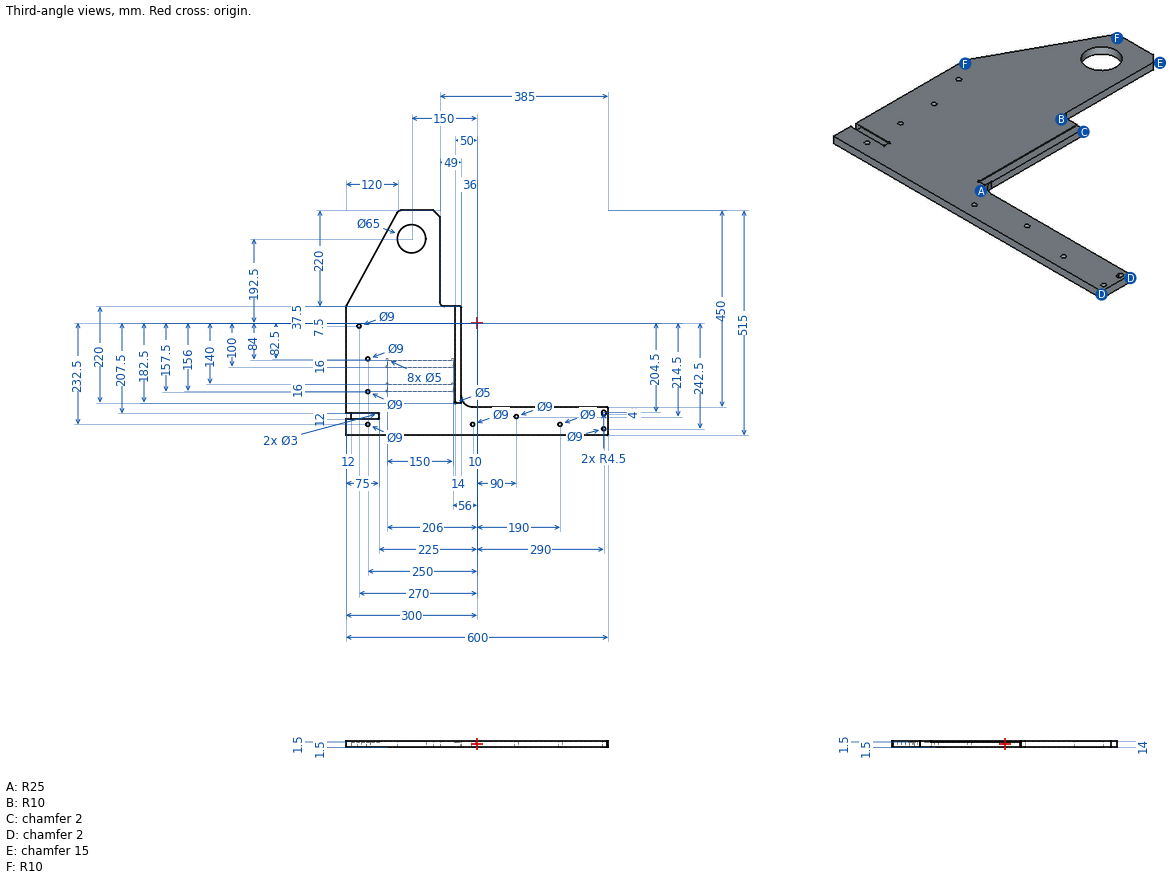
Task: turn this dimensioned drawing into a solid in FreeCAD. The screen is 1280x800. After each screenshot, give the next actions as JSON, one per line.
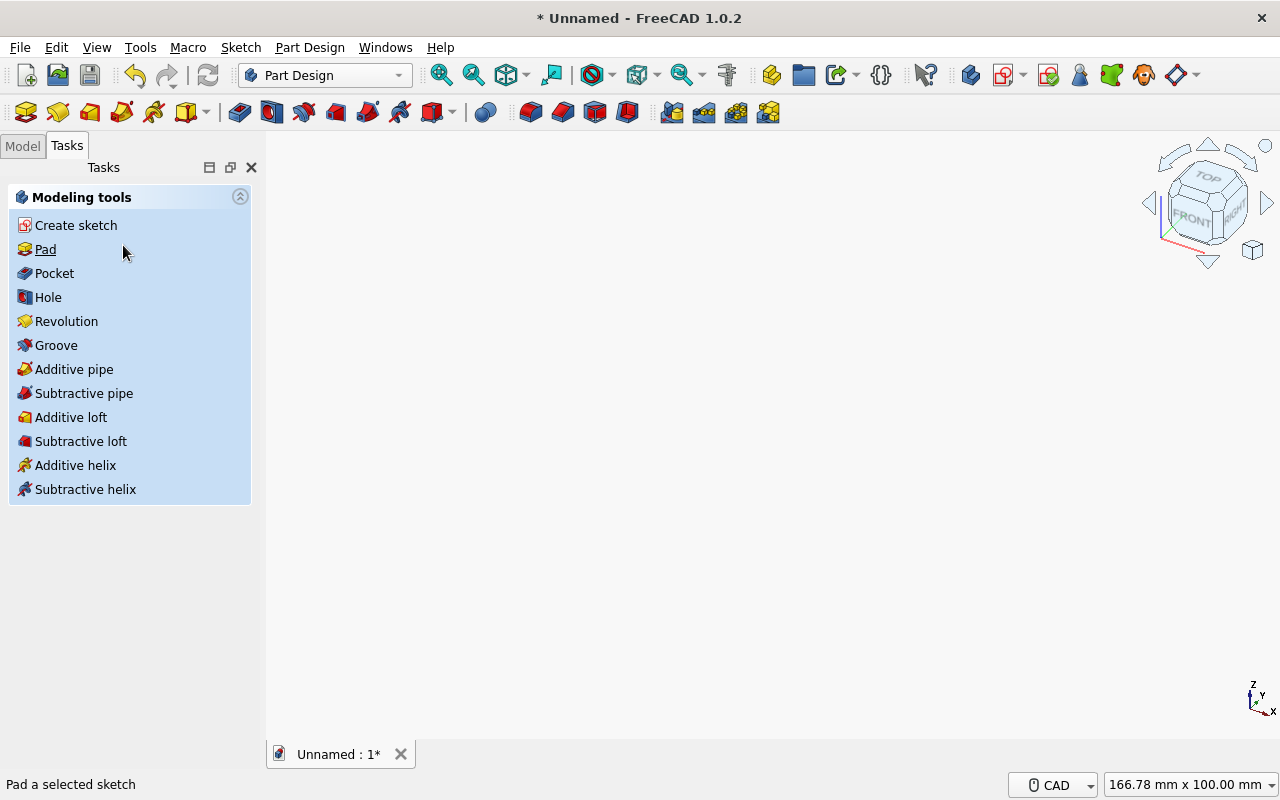
{"action": "left_click", "coordinate": [26, 112]}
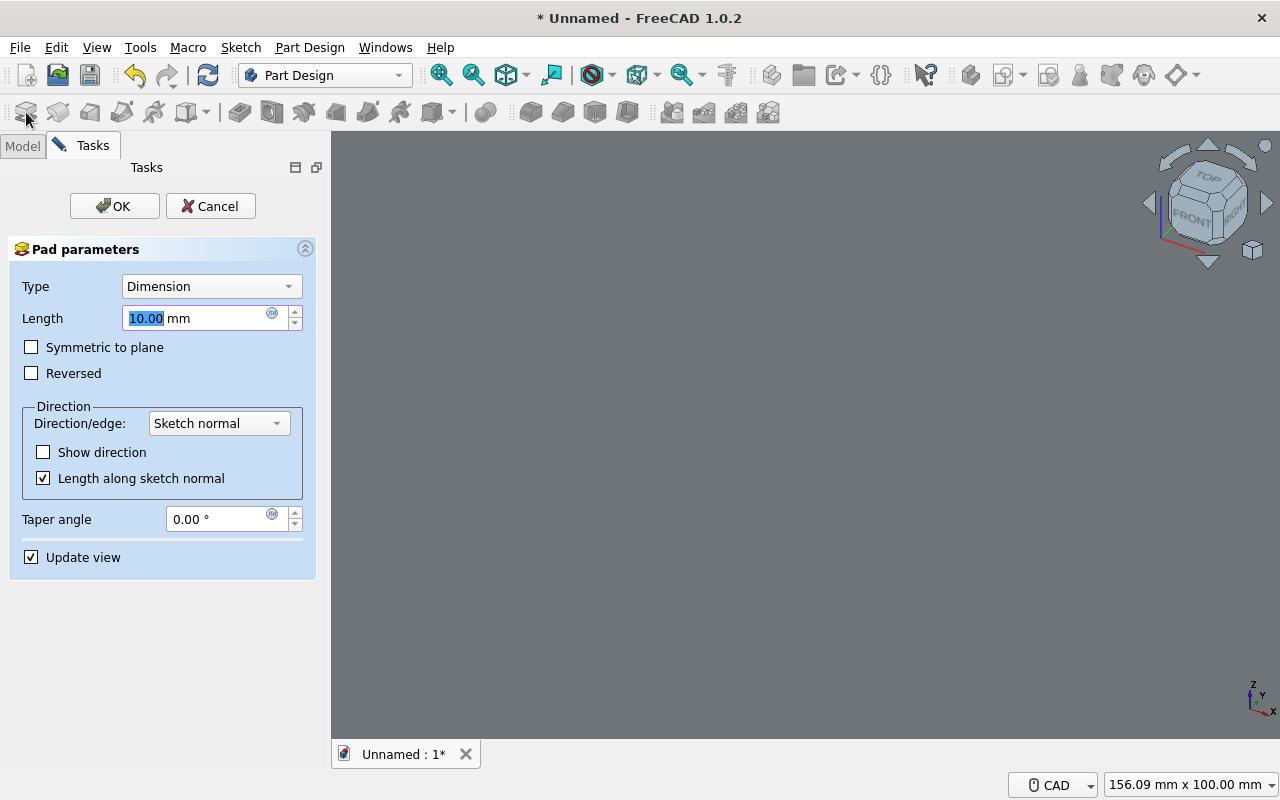
{"action": "type", "text": "14"}
{"action": "key", "text": "Tab"}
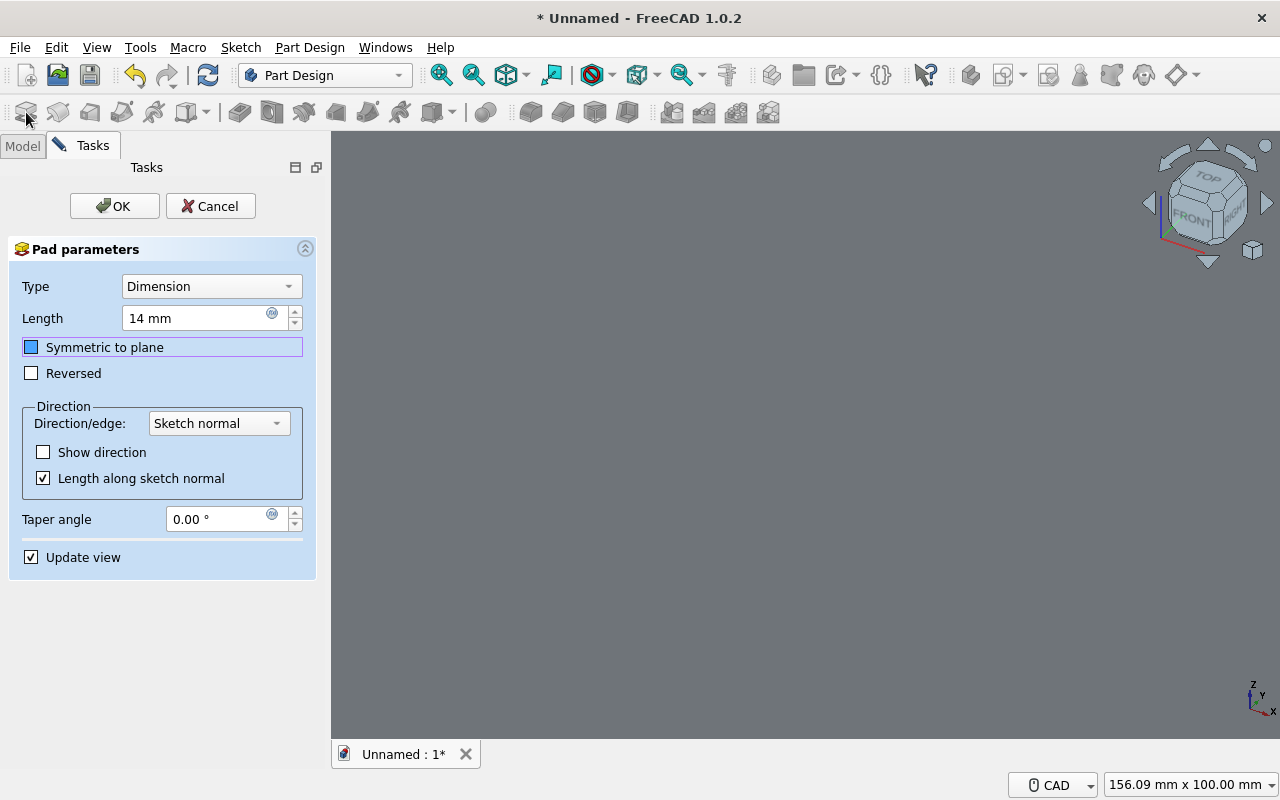
{"action": "left_click", "coordinate": [30, 347]}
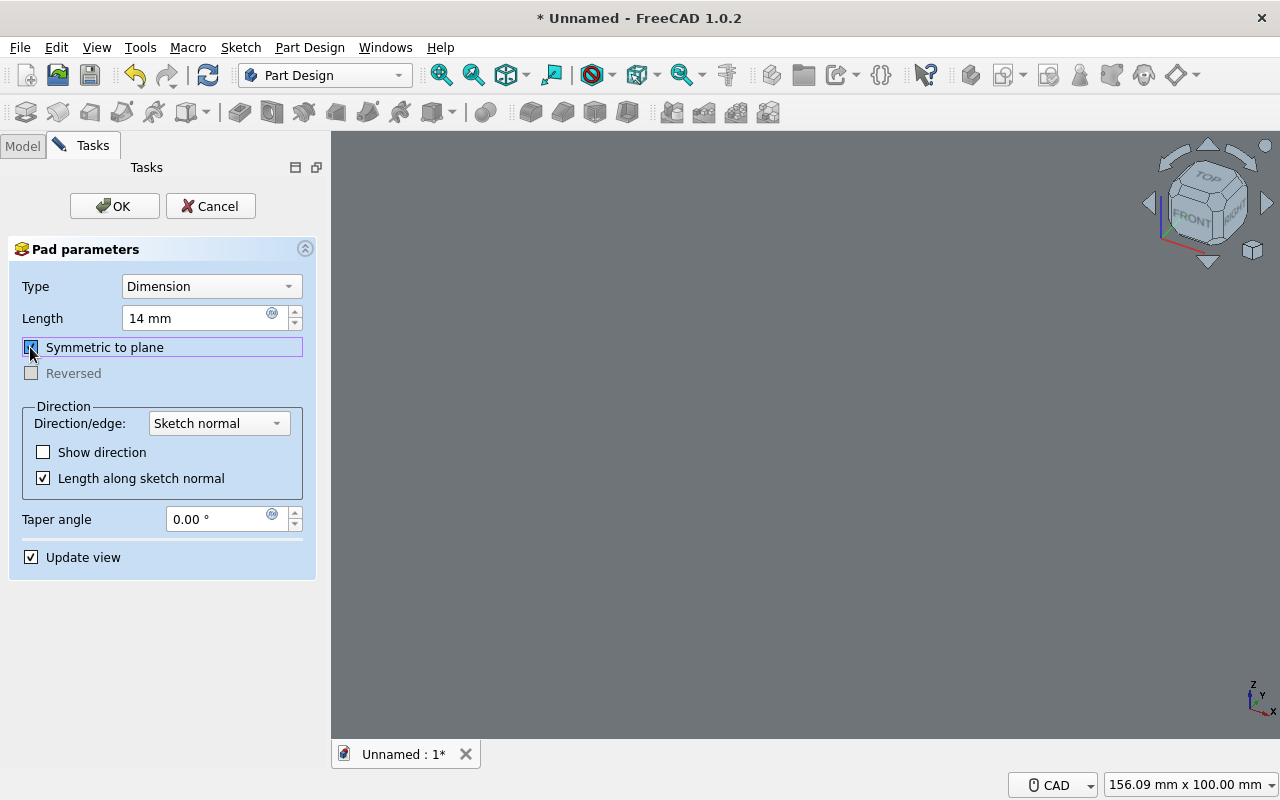
{"action": "left_click", "coordinate": [115, 206]}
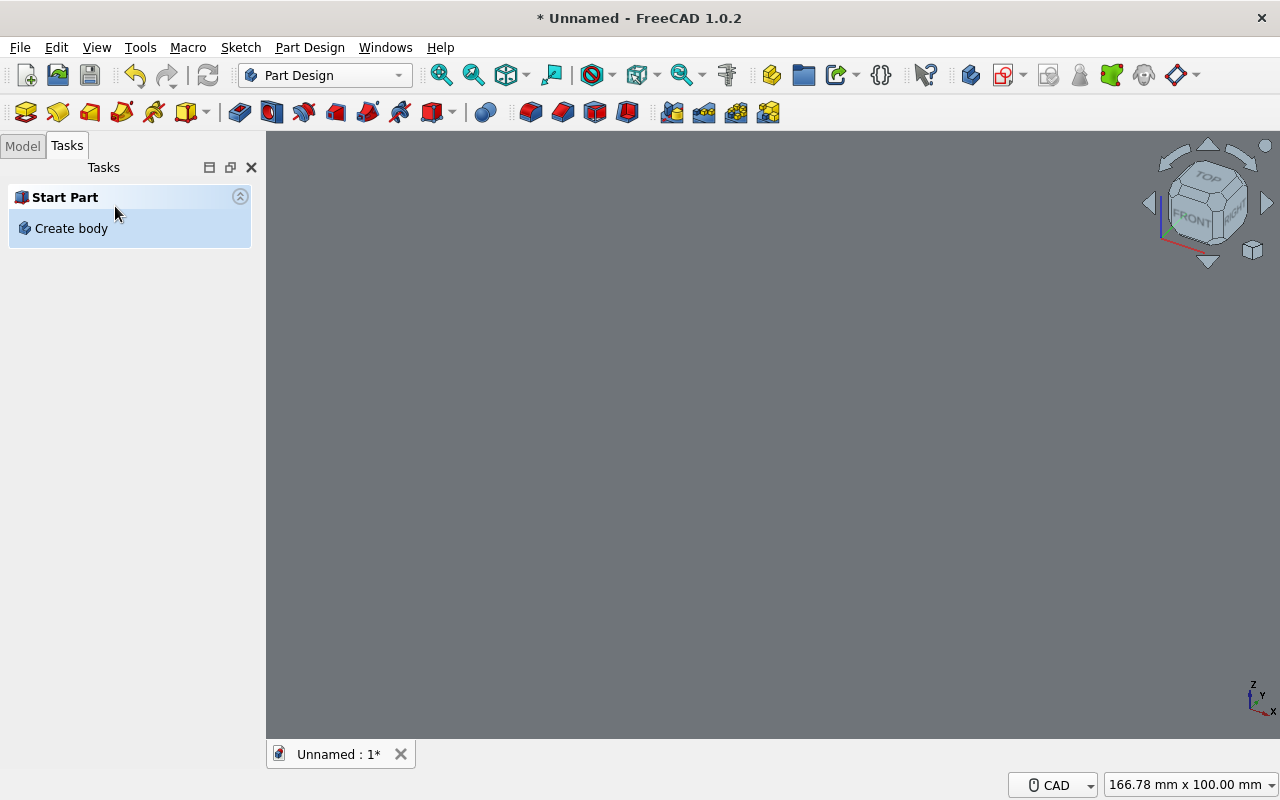
{"action": "left_click", "coordinate": [442, 76]}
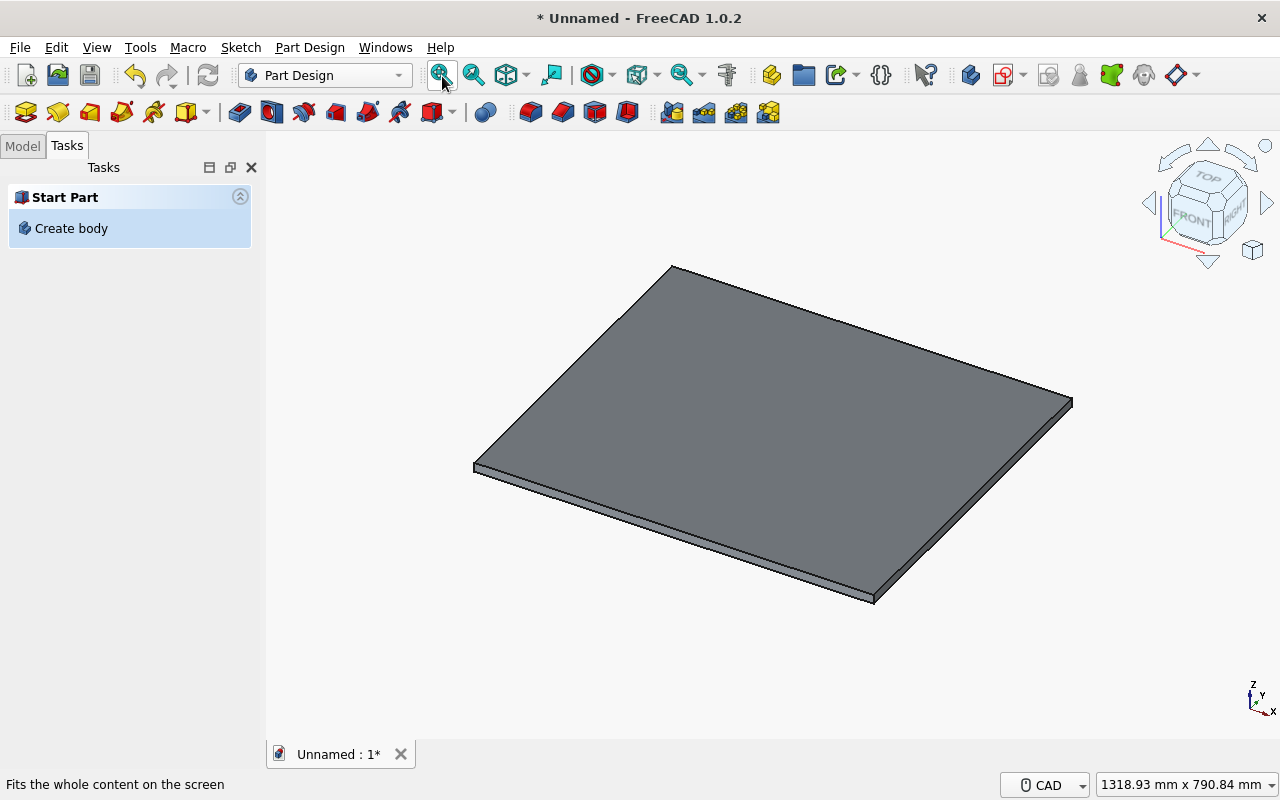
{"action": "left_click", "coordinate": [773, 430]}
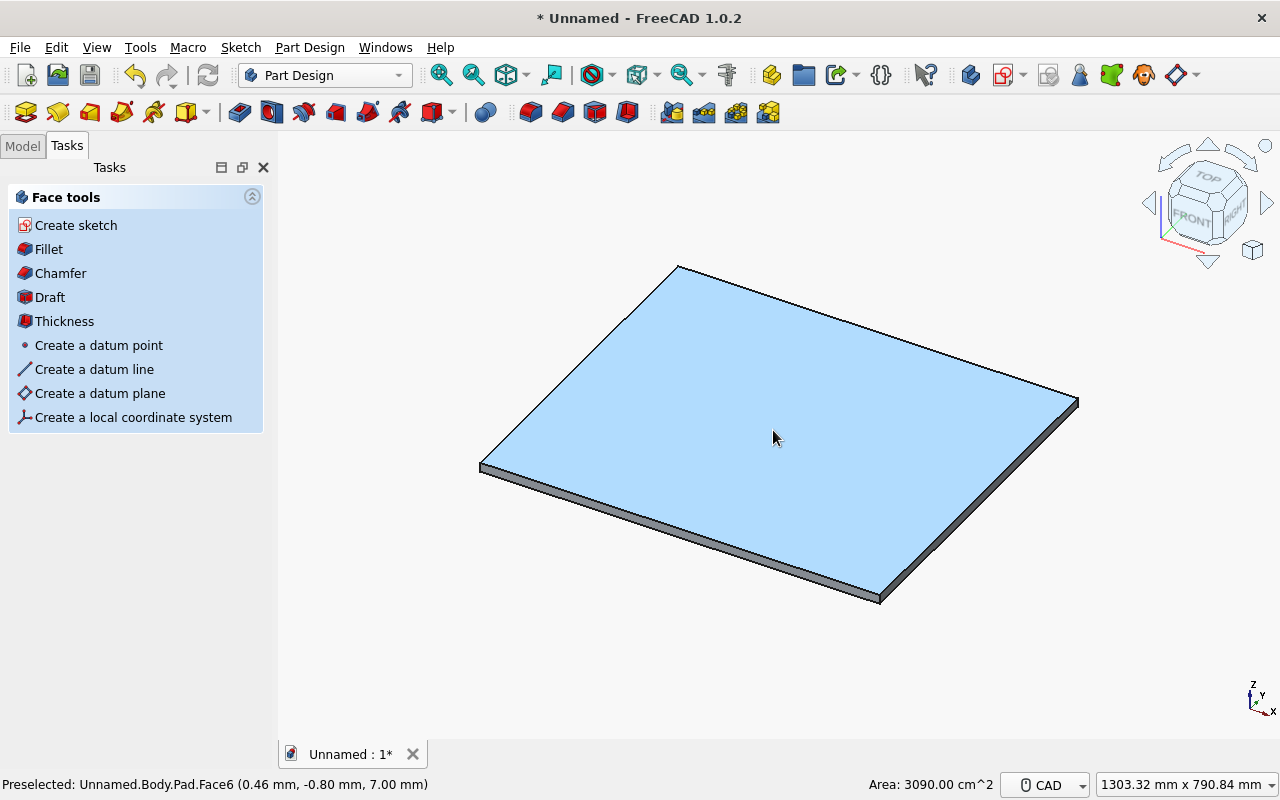
{"action": "left_click", "coordinate": [1004, 76]}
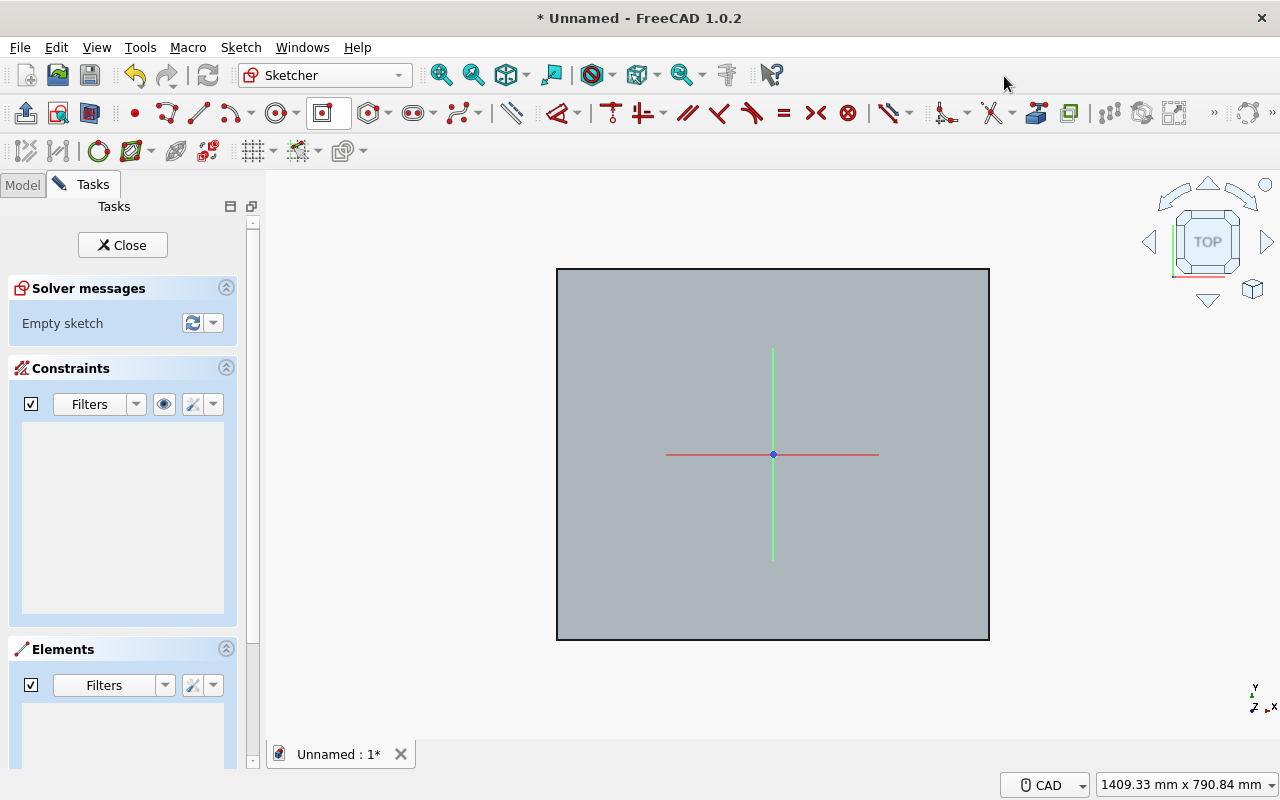
{"action": "scroll", "coordinate": [659, 294], "scroll_direction": "up", "scroll_amount": 10}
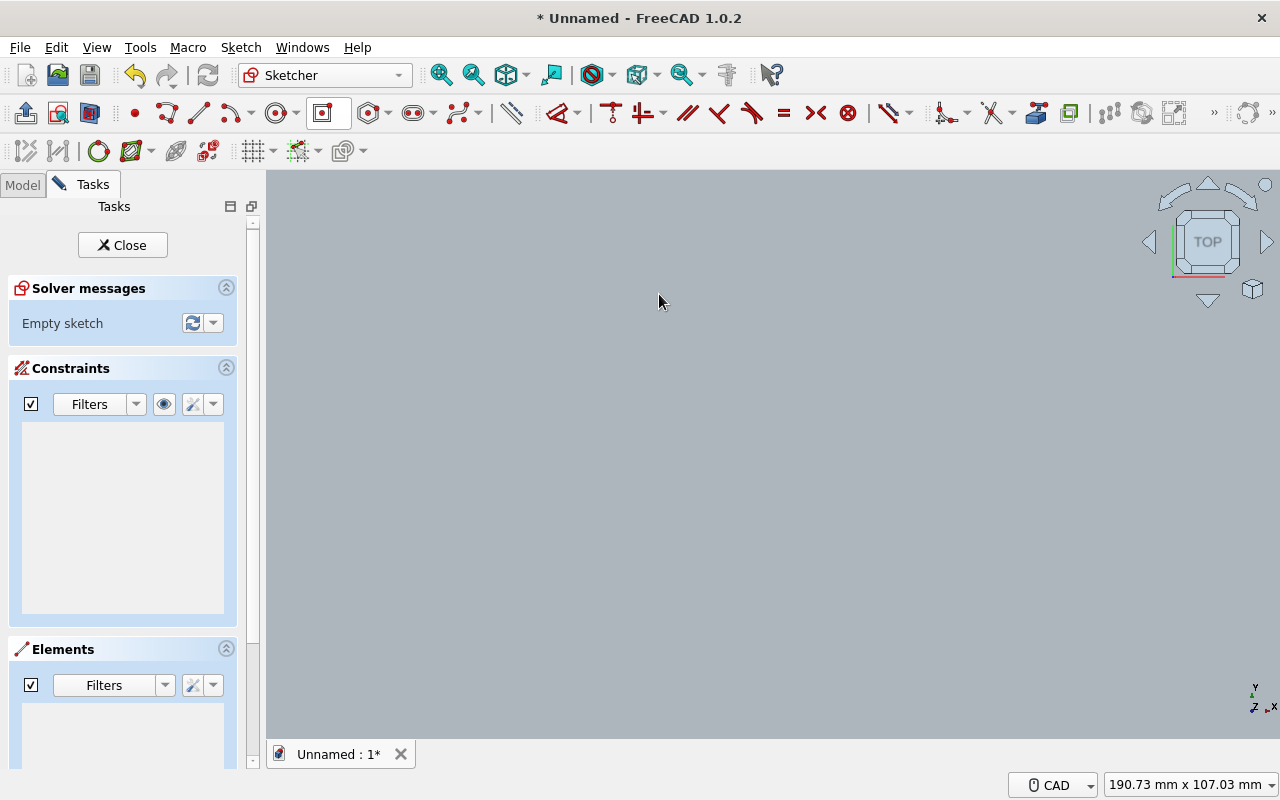
{"action": "left_click", "coordinate": [276, 114]}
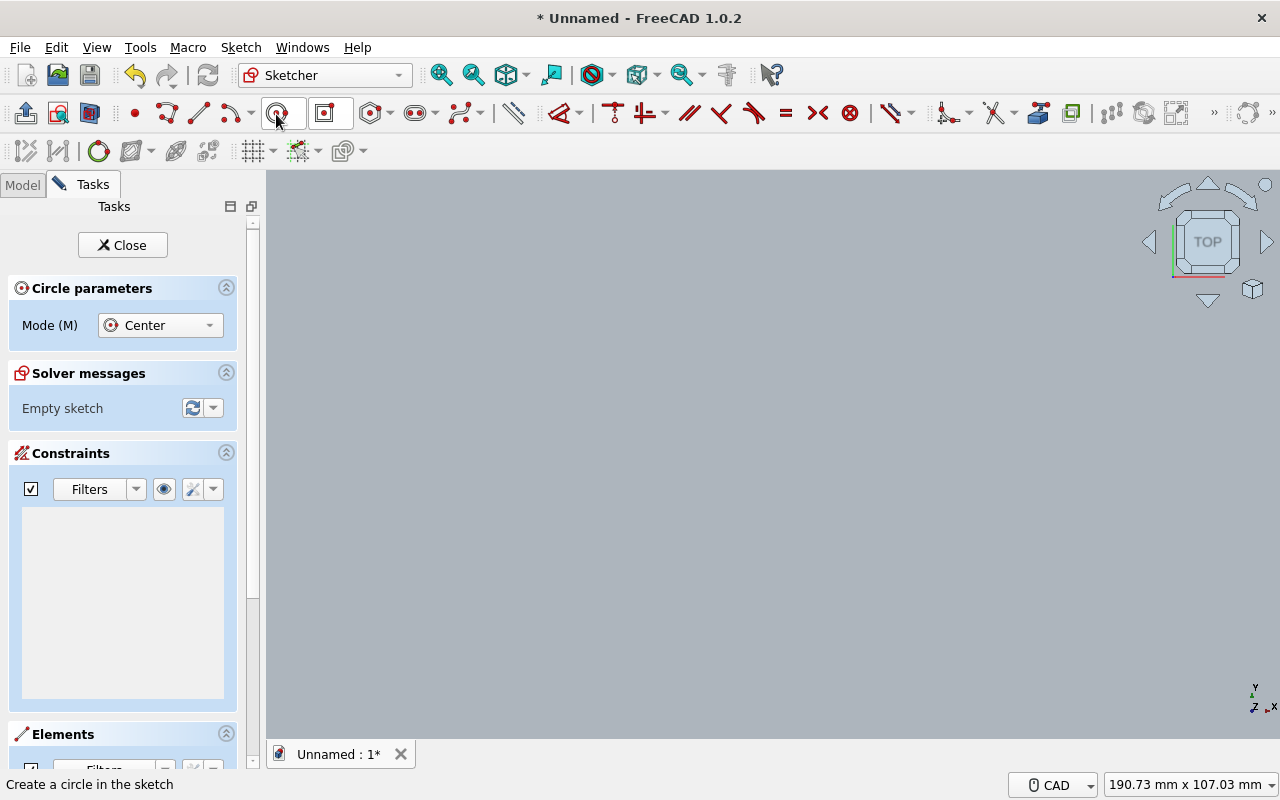
{"action": "left_click", "coordinate": [701, 455]}
{"action": "mouse_move", "coordinate": [824, 333]}